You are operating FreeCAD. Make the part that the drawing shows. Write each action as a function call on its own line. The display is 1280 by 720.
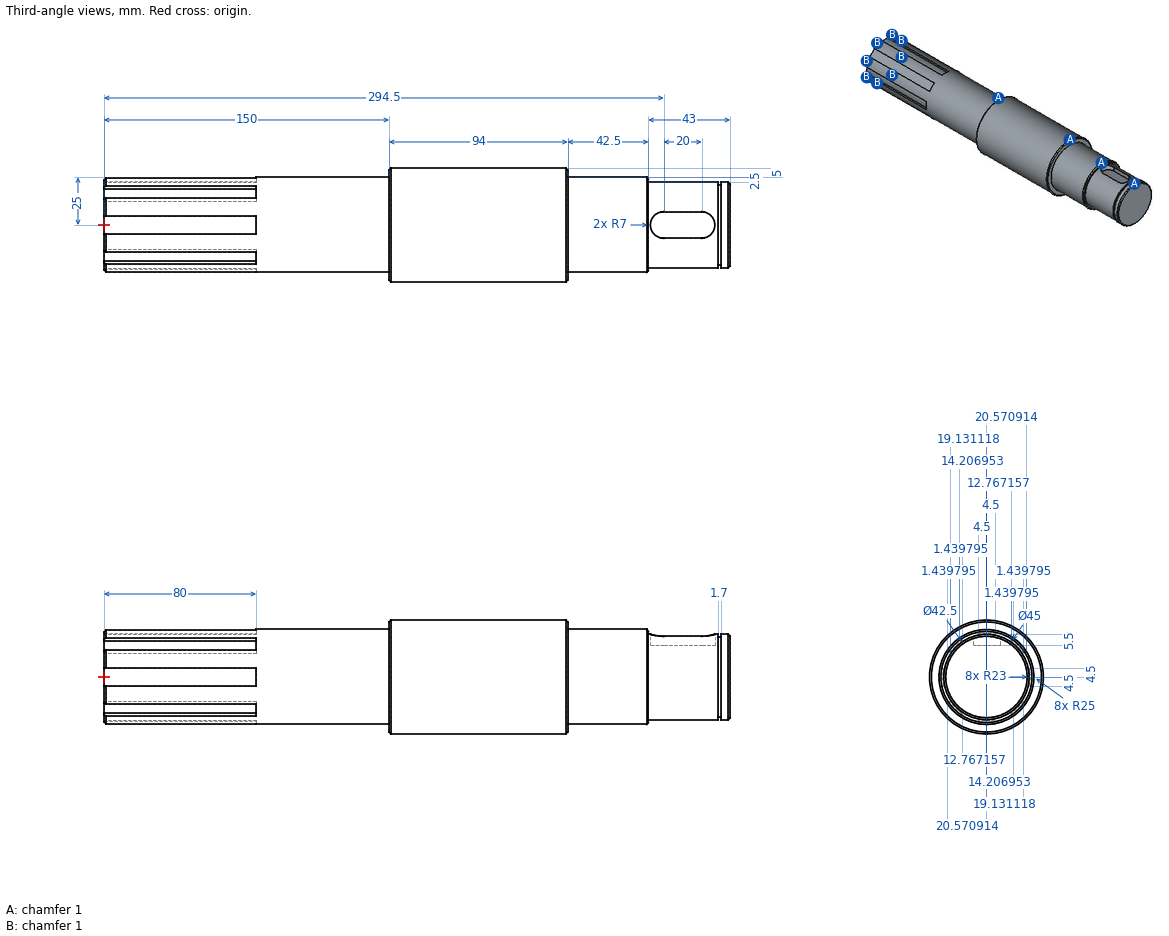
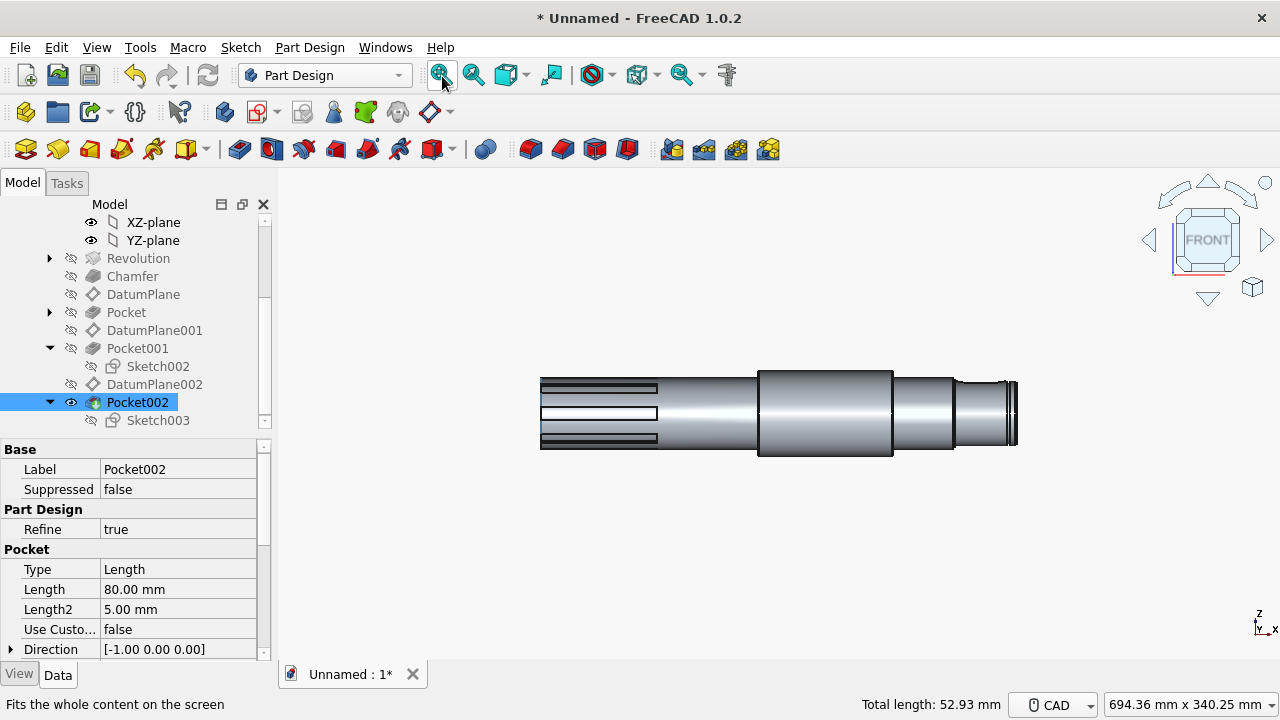
scroll(541, 446, up, 5)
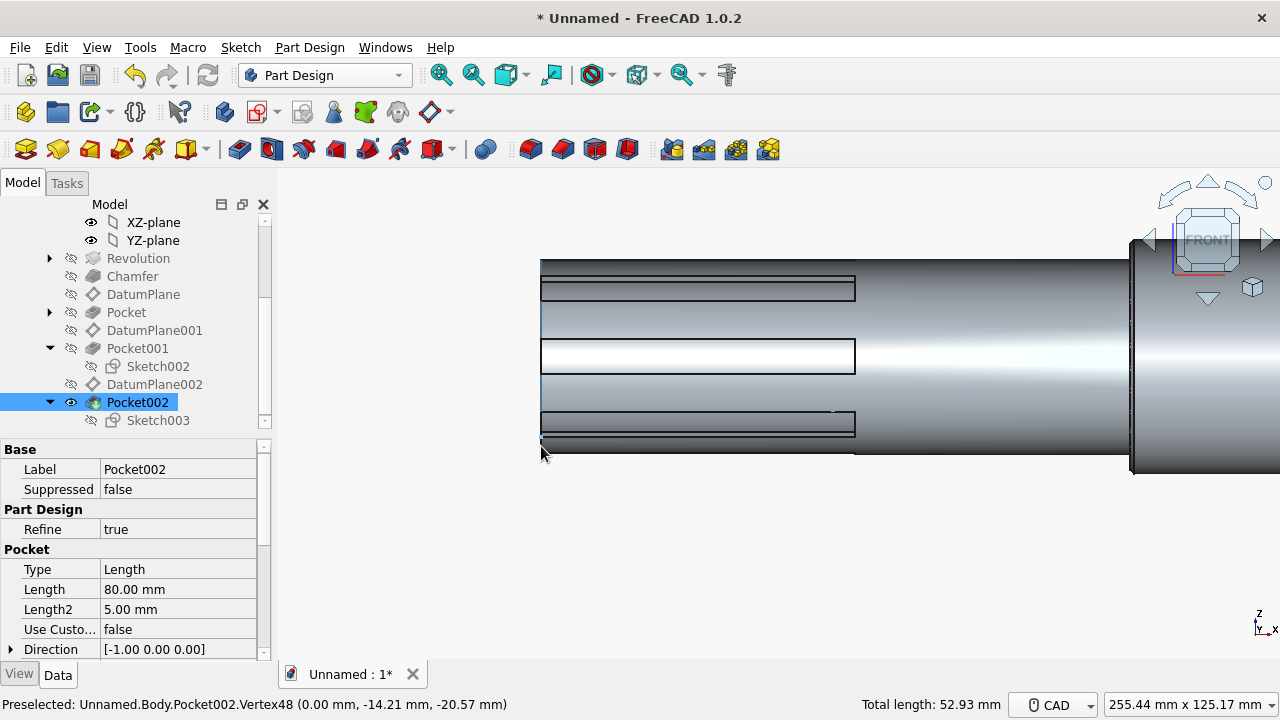
click(541, 443, ctrl)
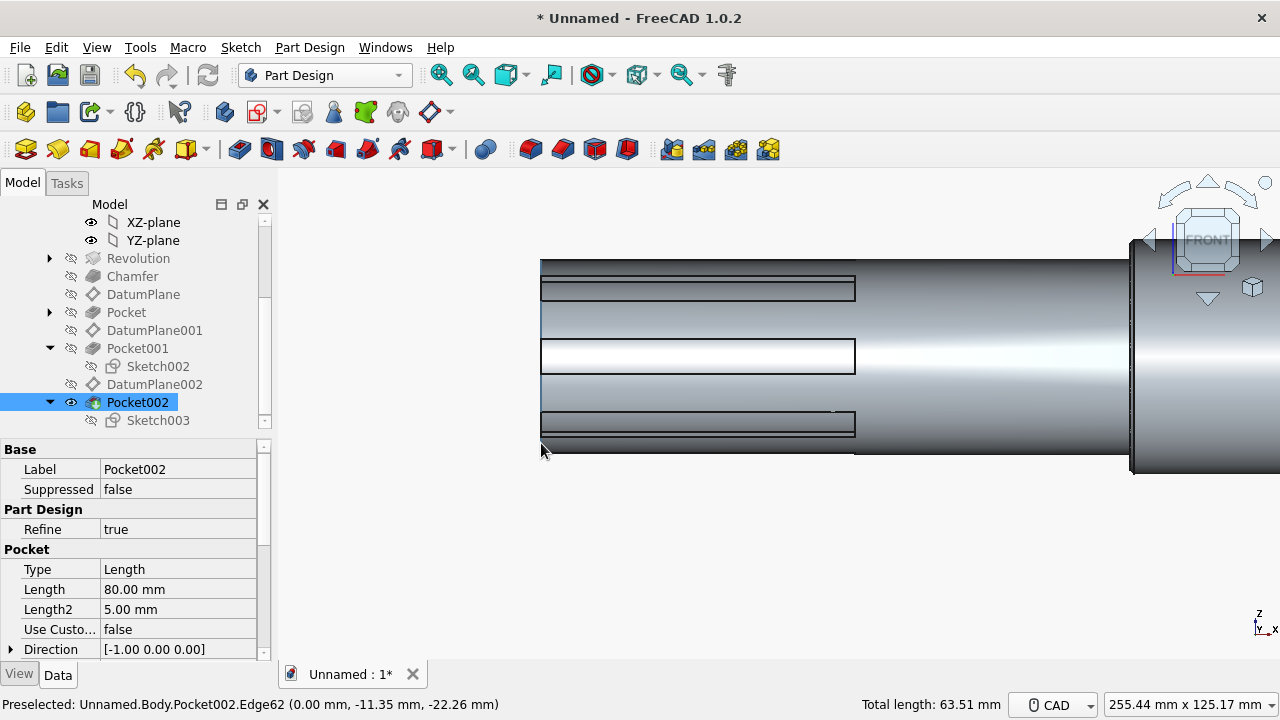
click(442, 76)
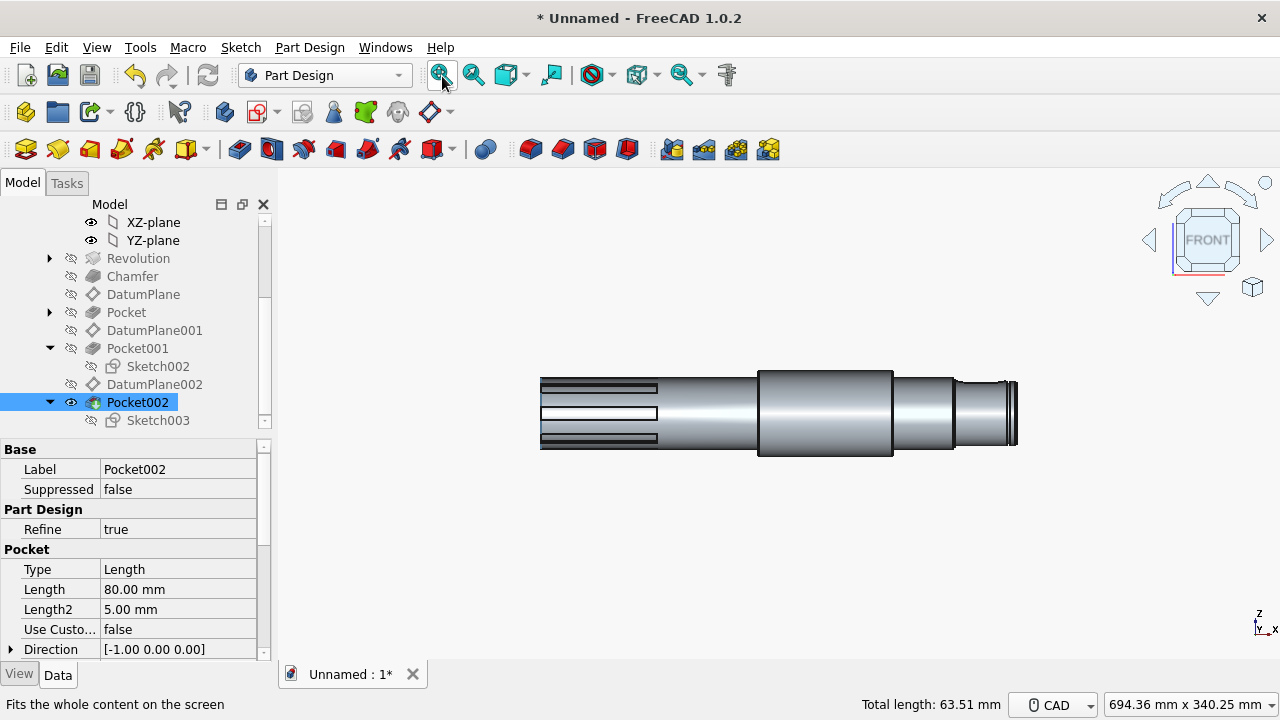
key(3)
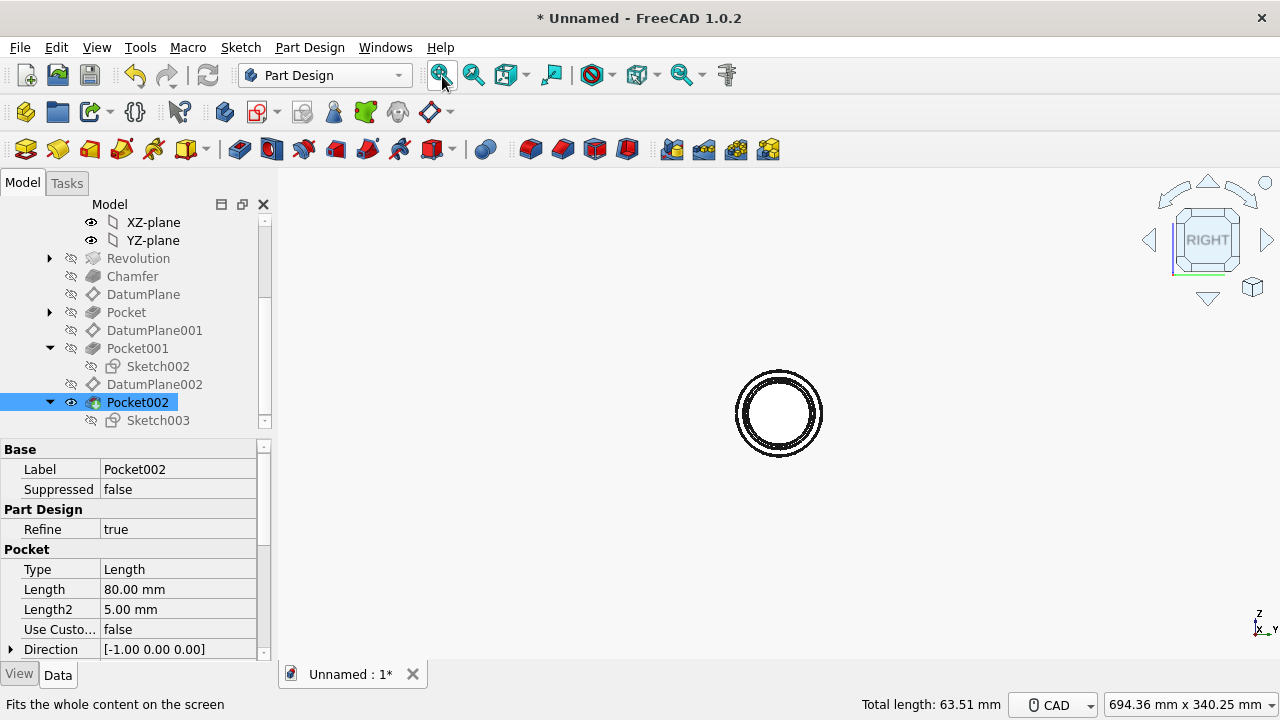
click(442, 76)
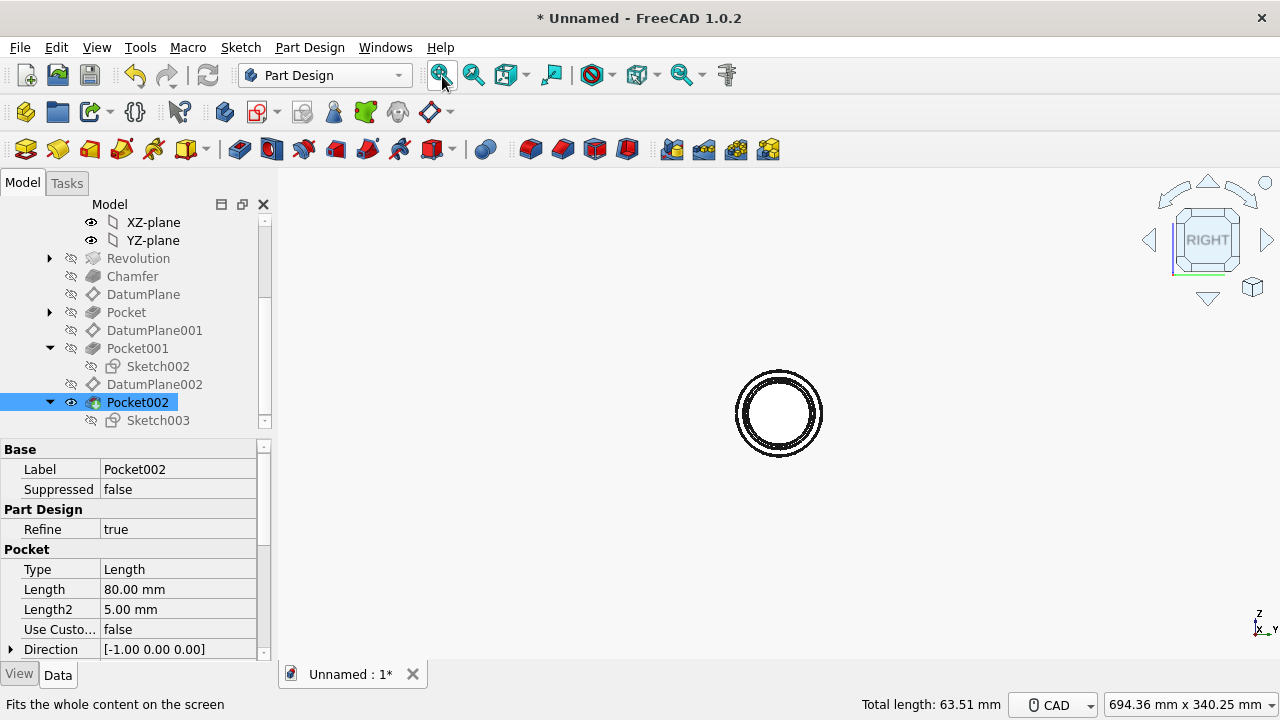
scroll(793, 446, up, 5)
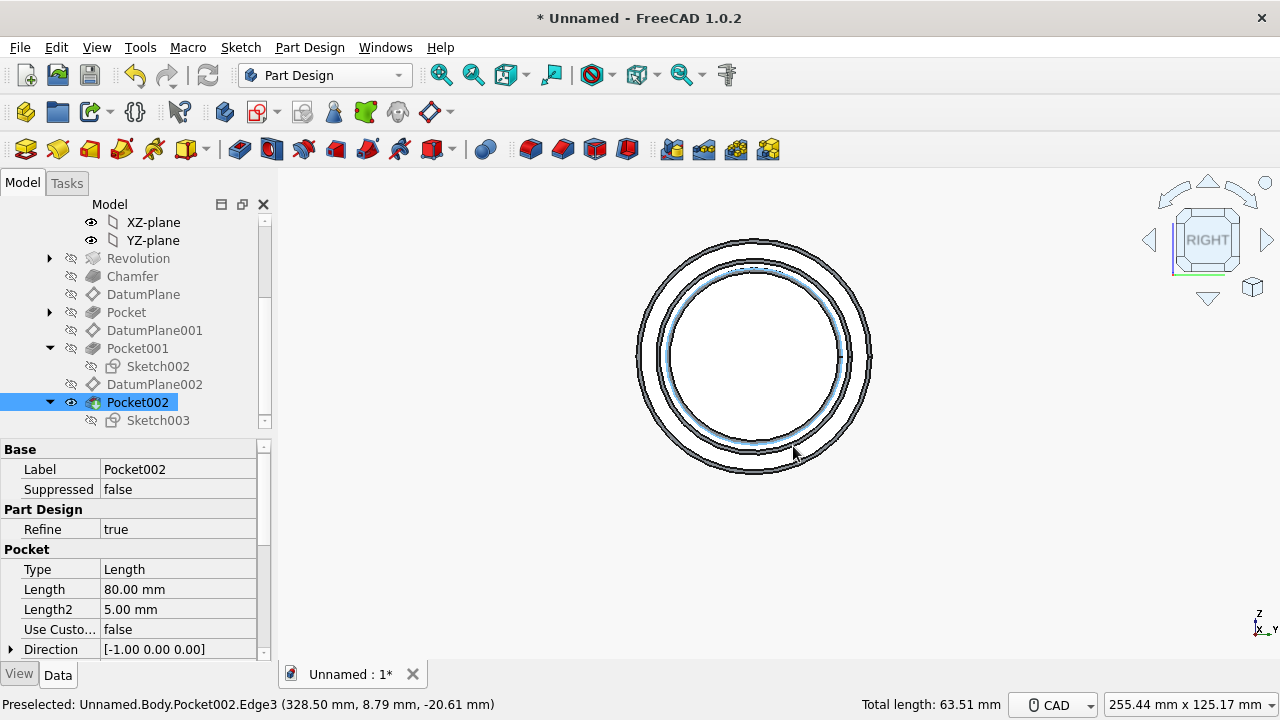
click(442, 76)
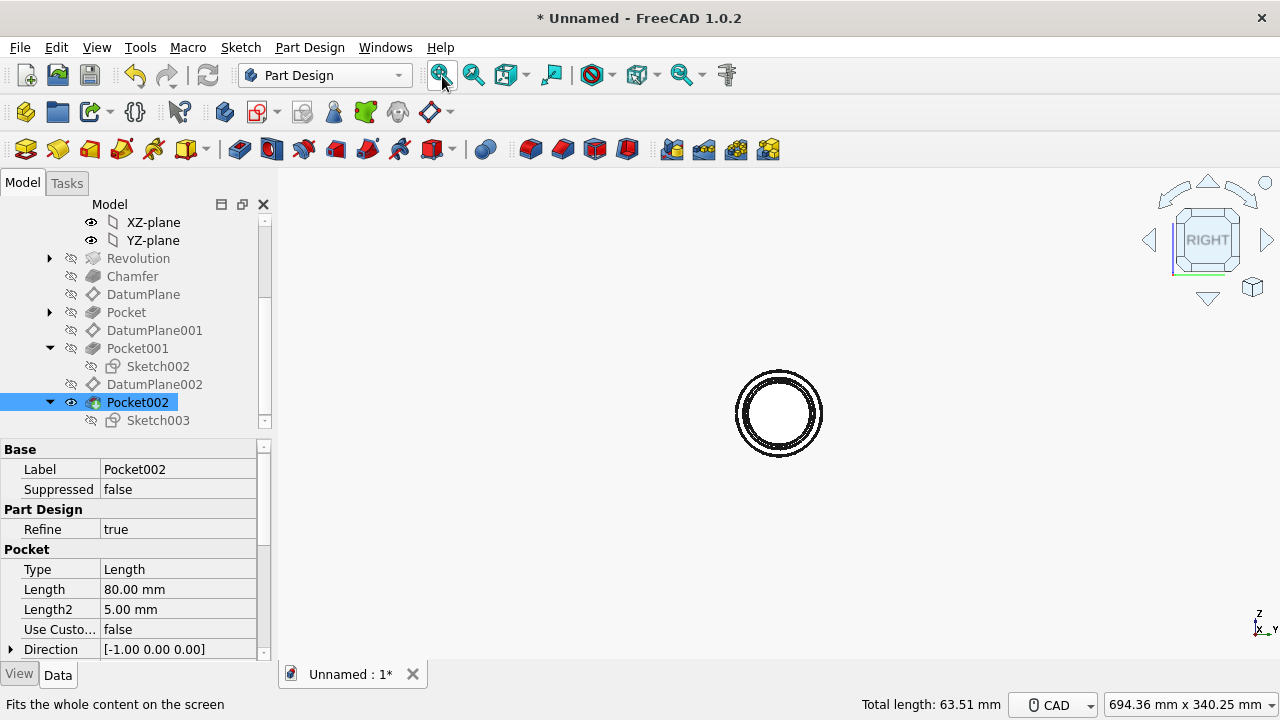
key(5)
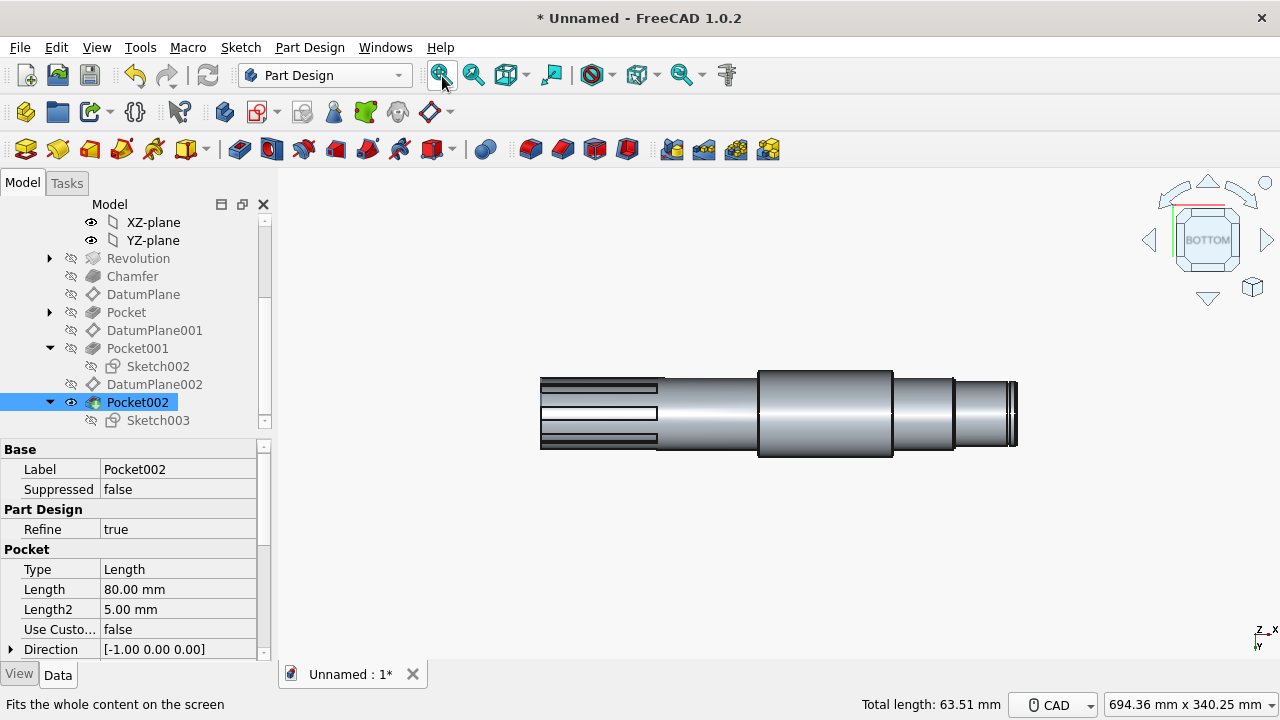
click(541, 426, ctrl)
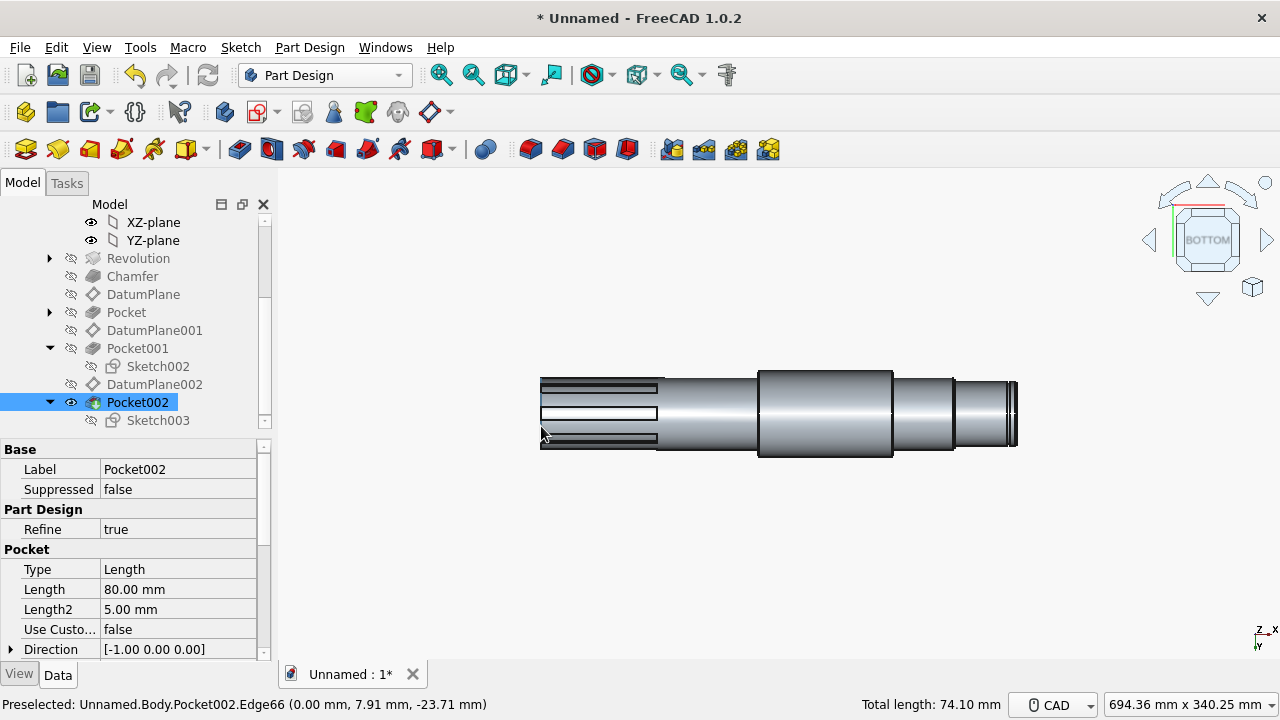
scroll(541, 446, up, 5)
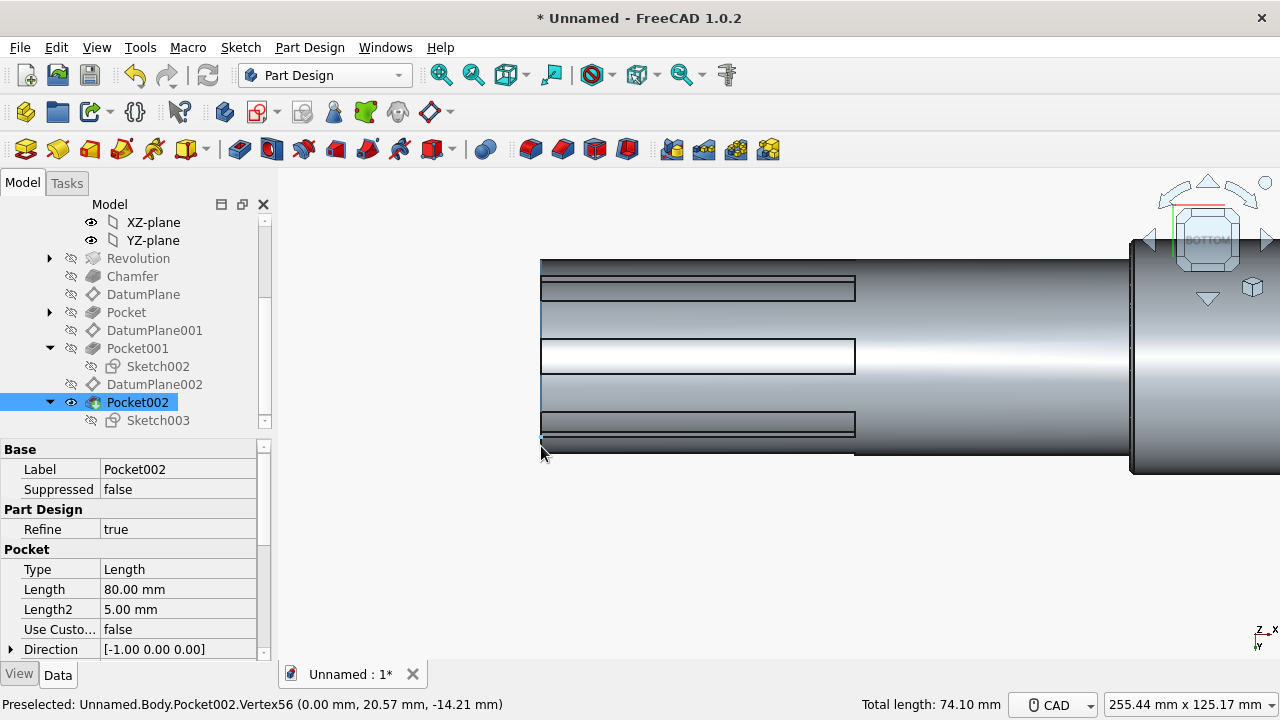
click(541, 443, ctrl)